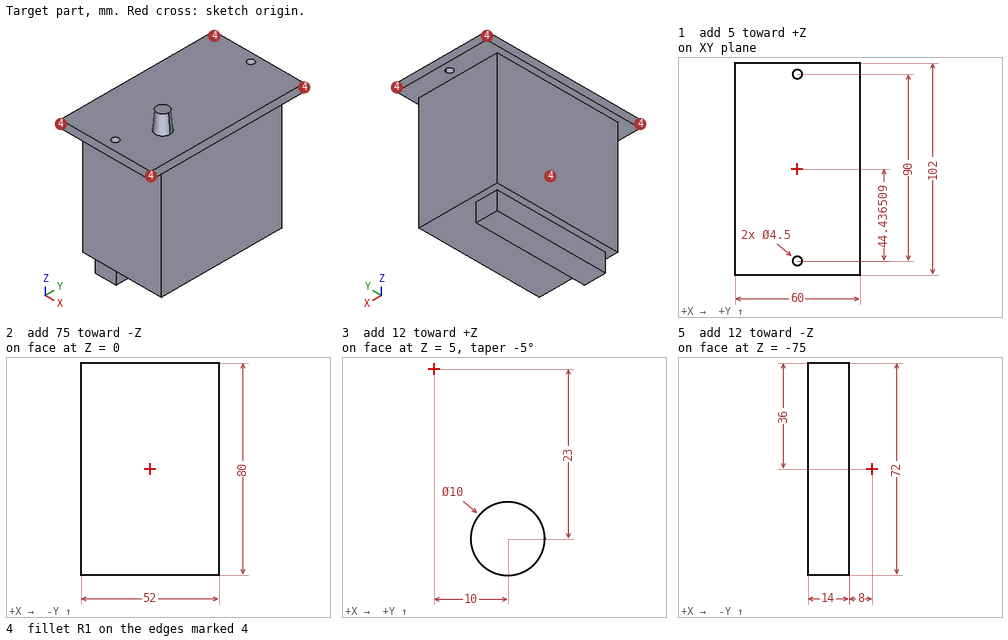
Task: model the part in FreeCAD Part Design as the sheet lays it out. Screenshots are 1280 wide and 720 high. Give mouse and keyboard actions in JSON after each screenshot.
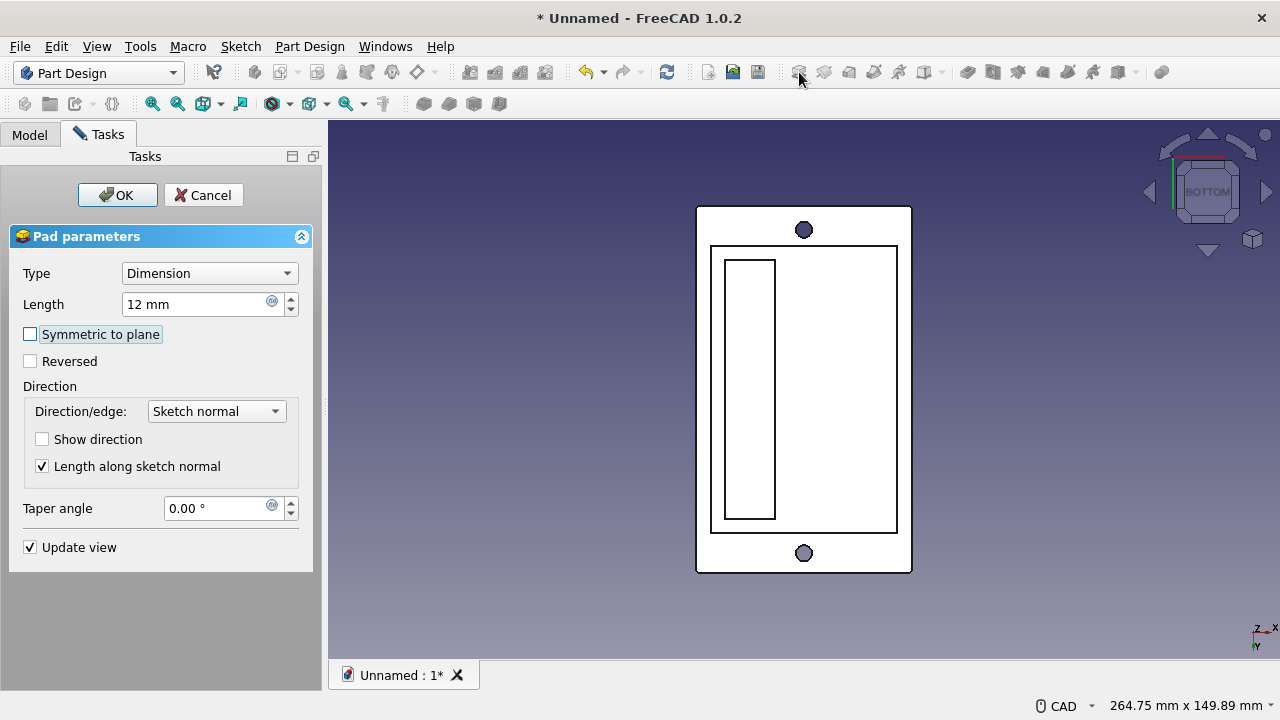
{"action": "left_click", "coordinate": [118, 195]}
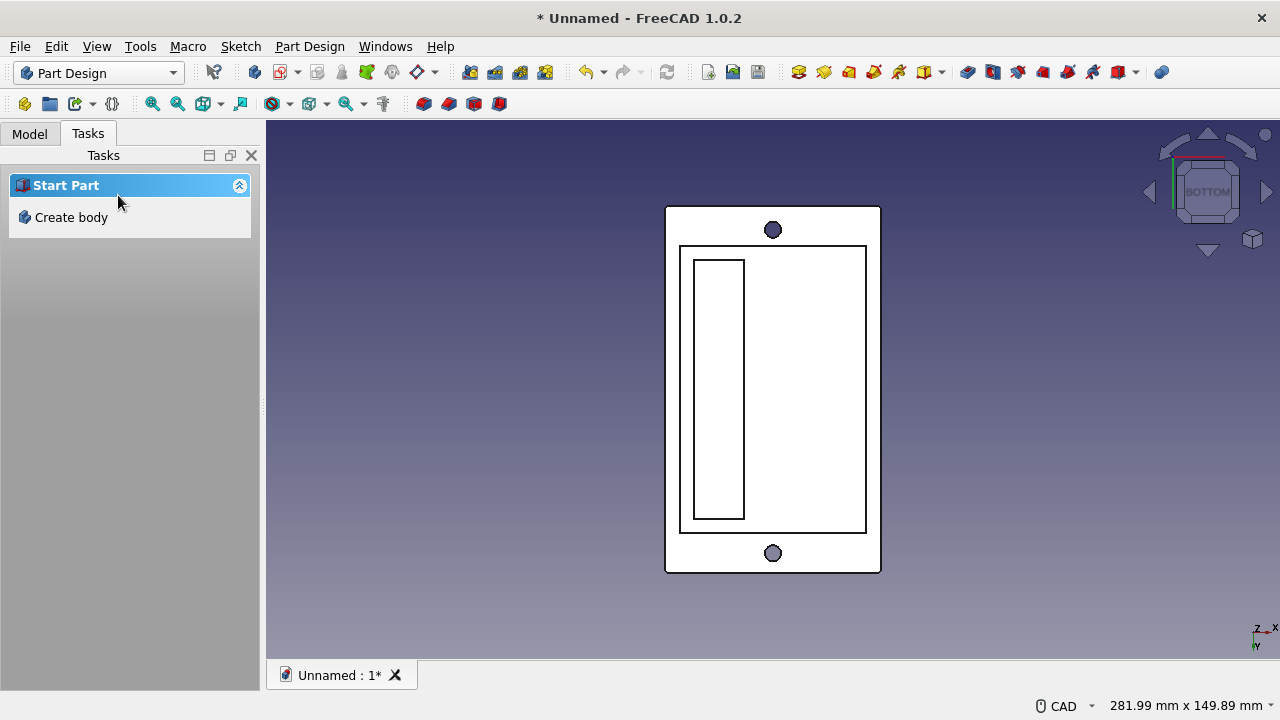
{"action": "key", "text": "0"}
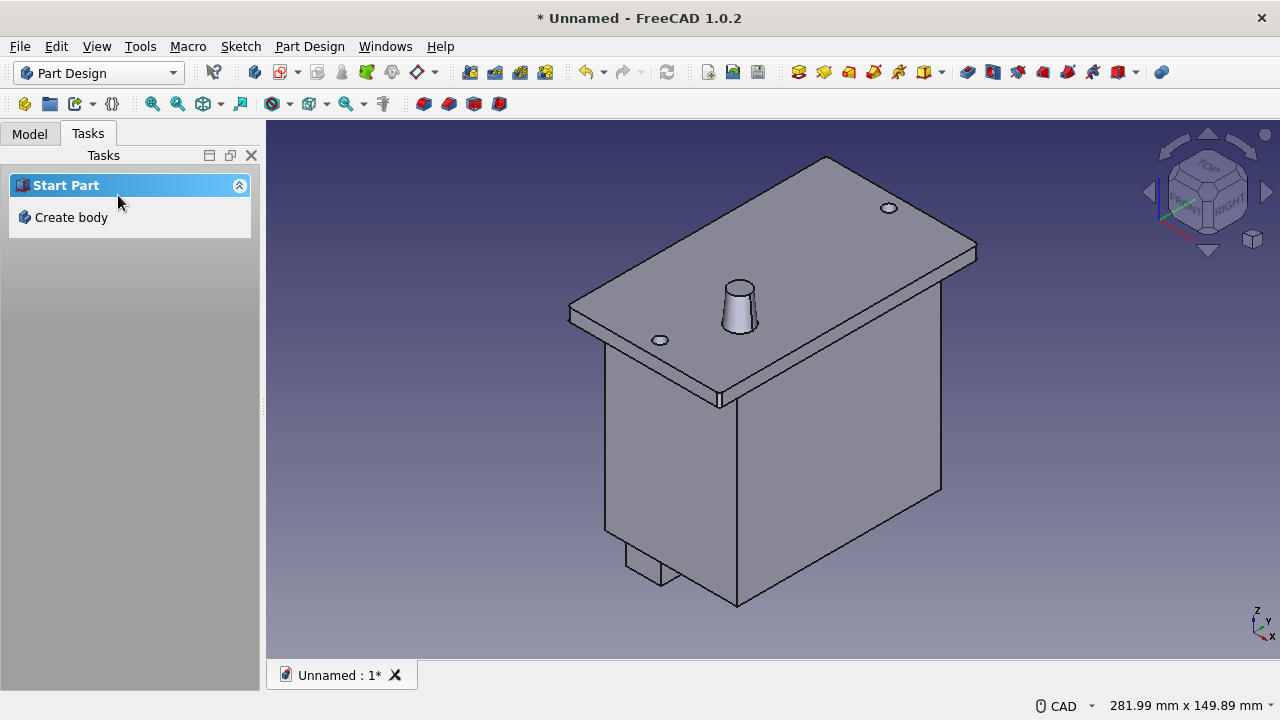
{"action": "key", "text": "v f"}